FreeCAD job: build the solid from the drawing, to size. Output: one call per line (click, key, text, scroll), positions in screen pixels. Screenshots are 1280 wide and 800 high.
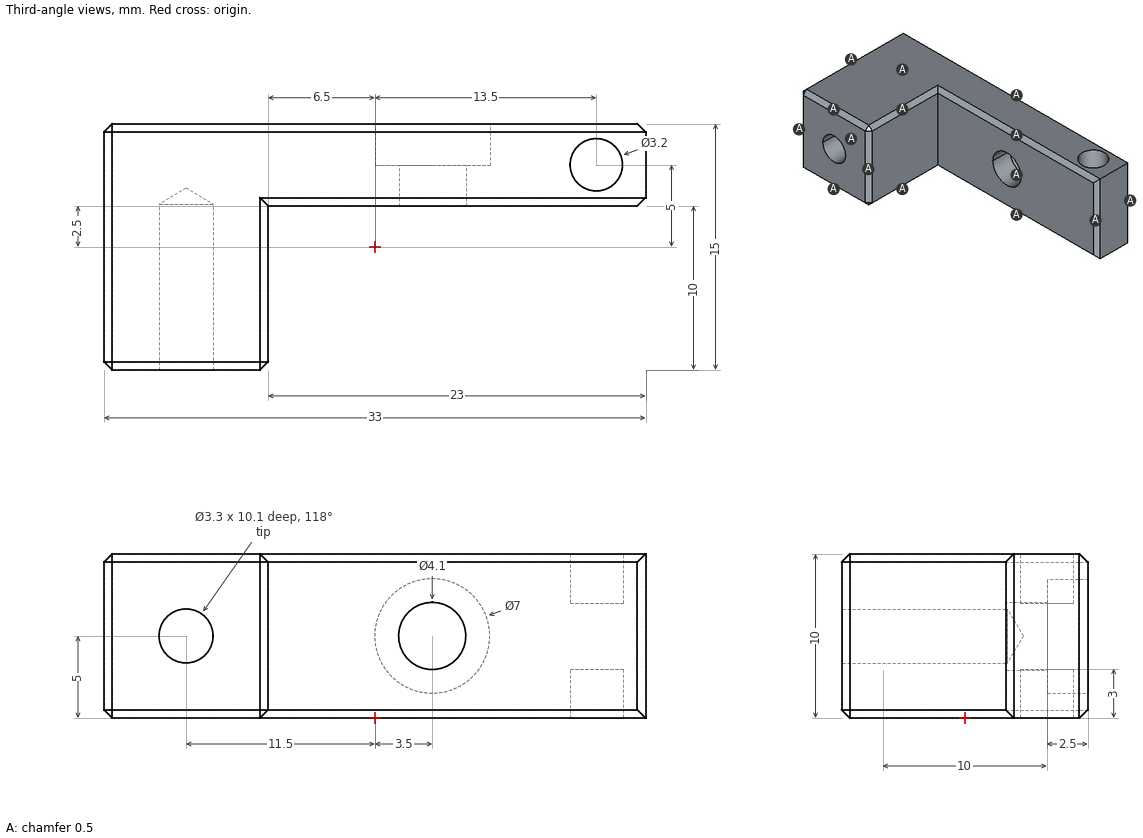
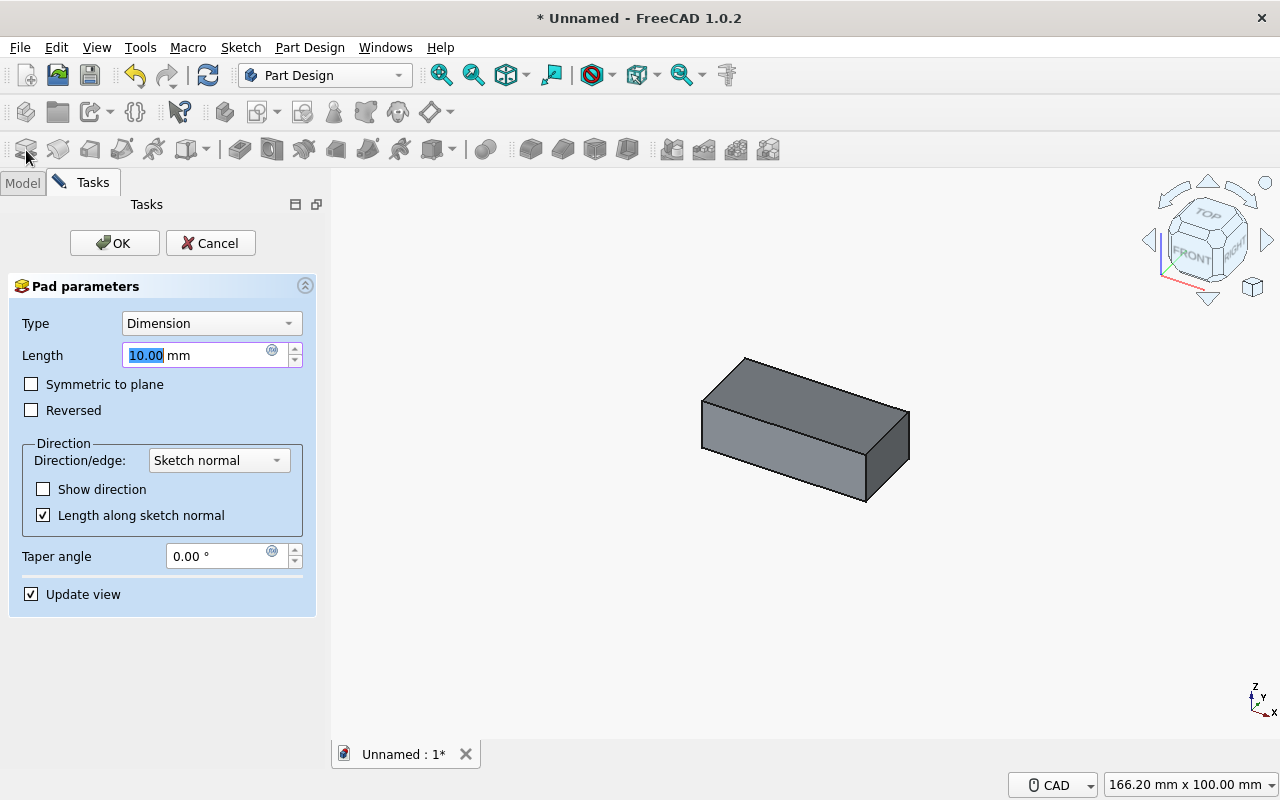
text(10)
key(Tab)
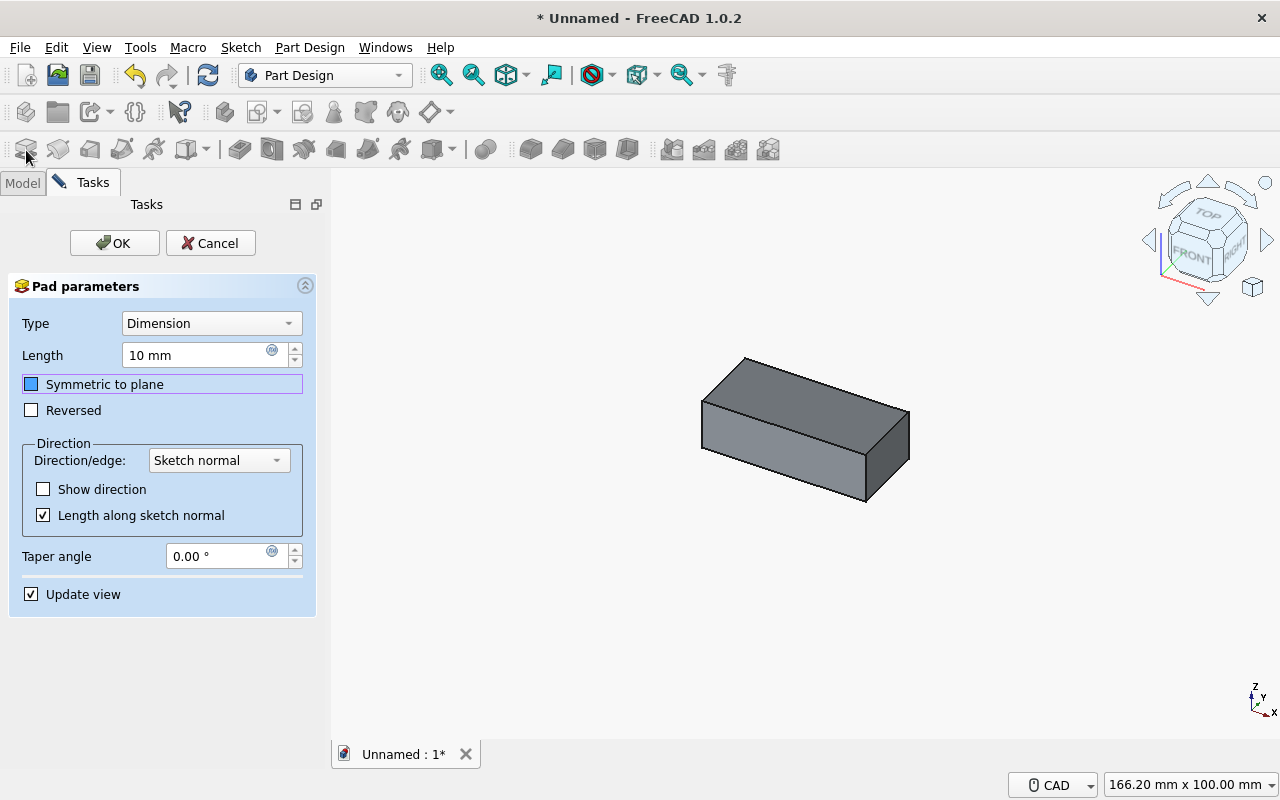
click(115, 243)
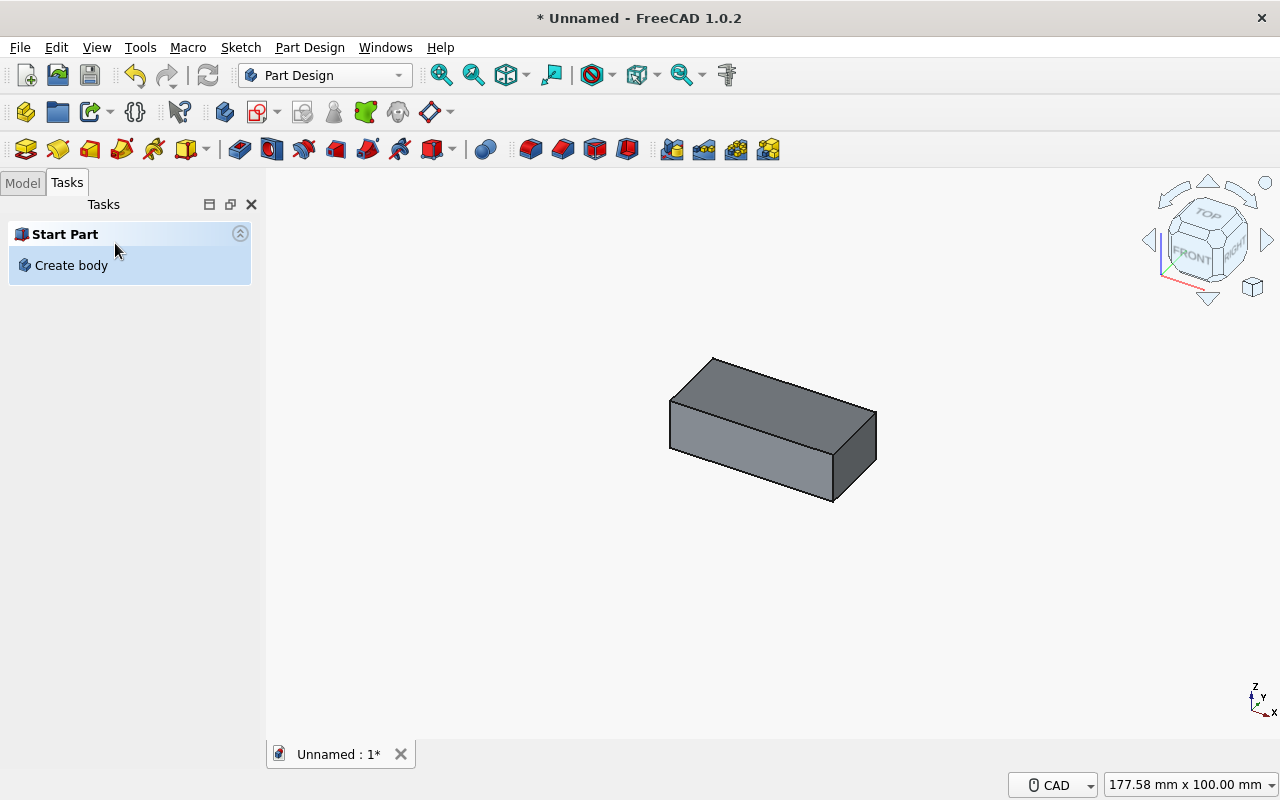
click(442, 76)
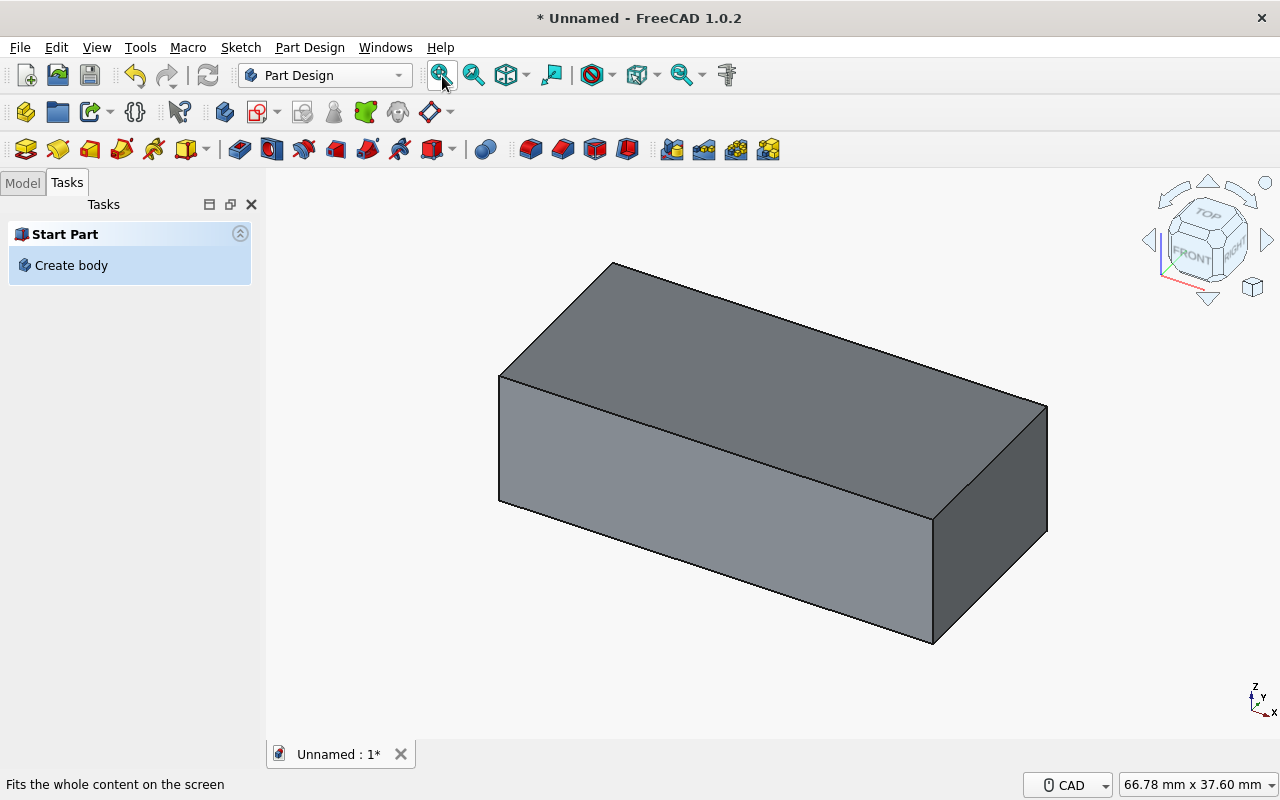
click(835, 411)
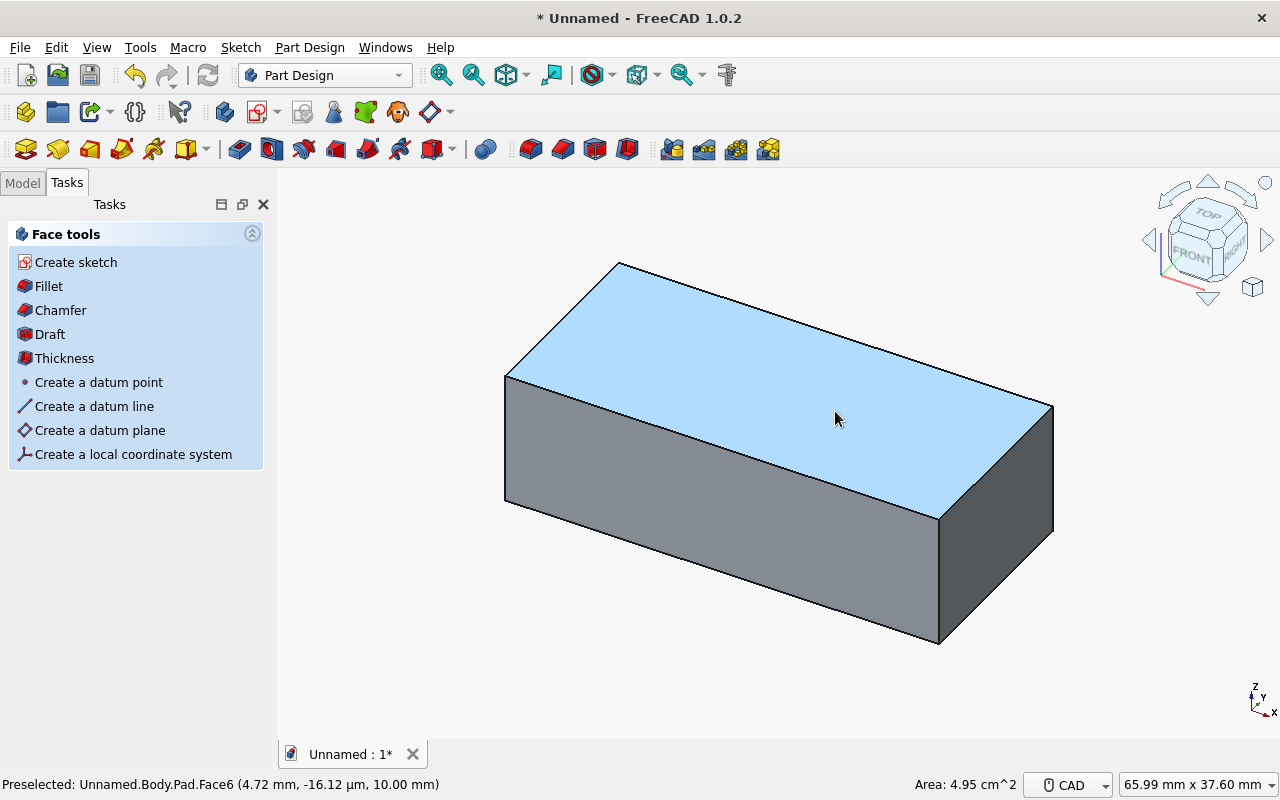
click(258, 112)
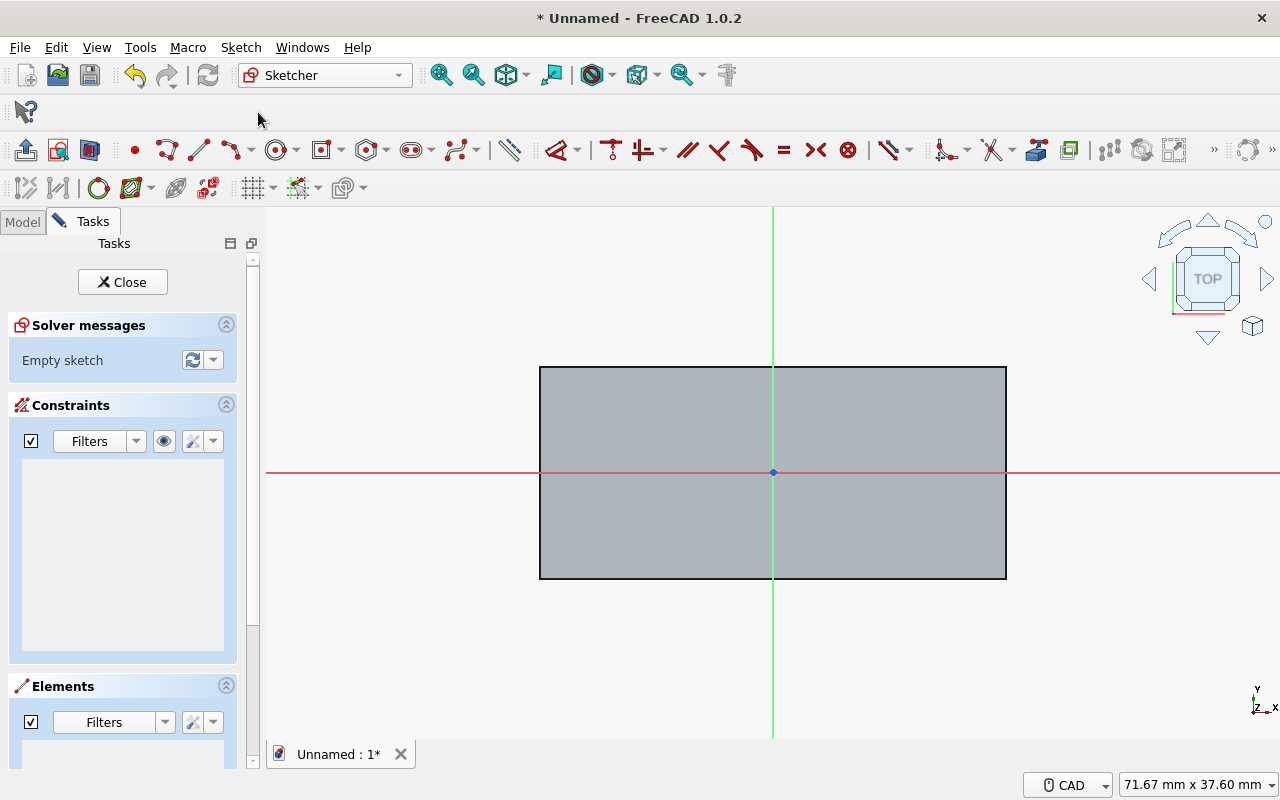
scroll(1013, 551, up, 3)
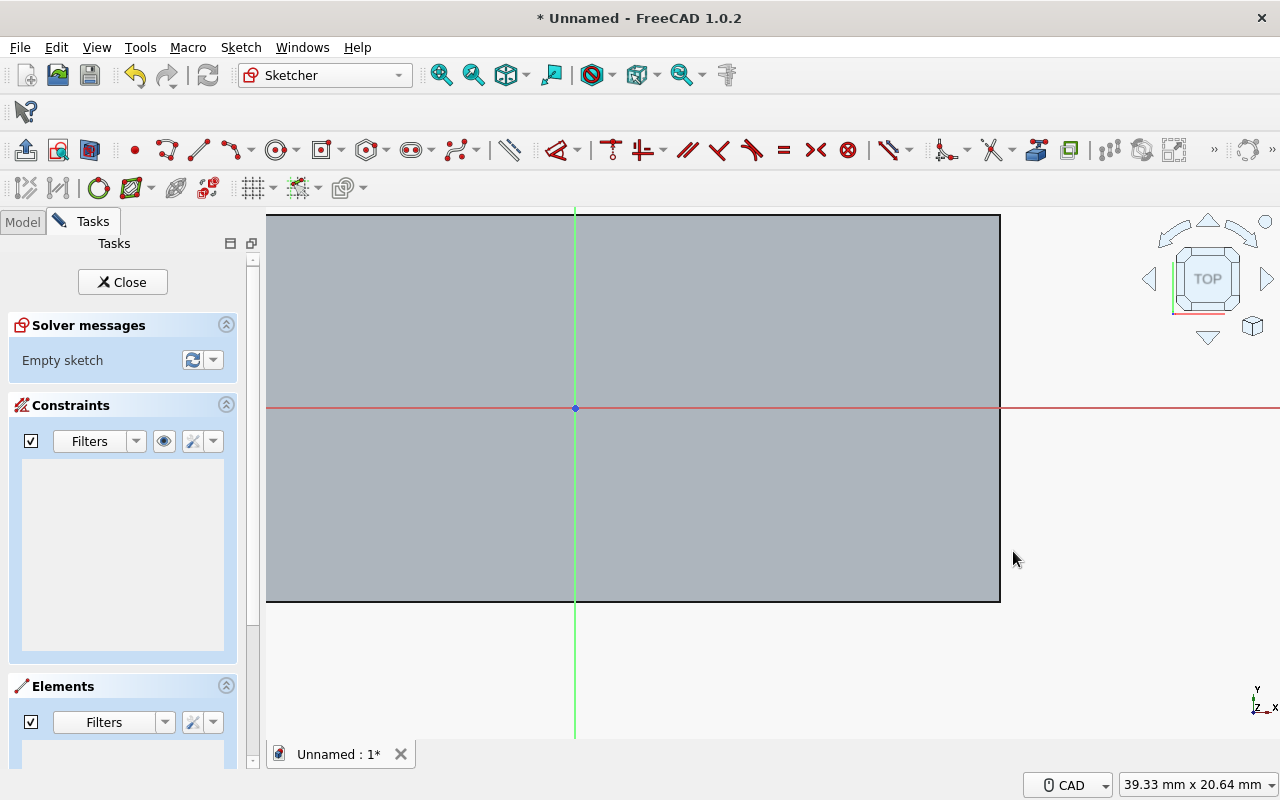
click(344, 150)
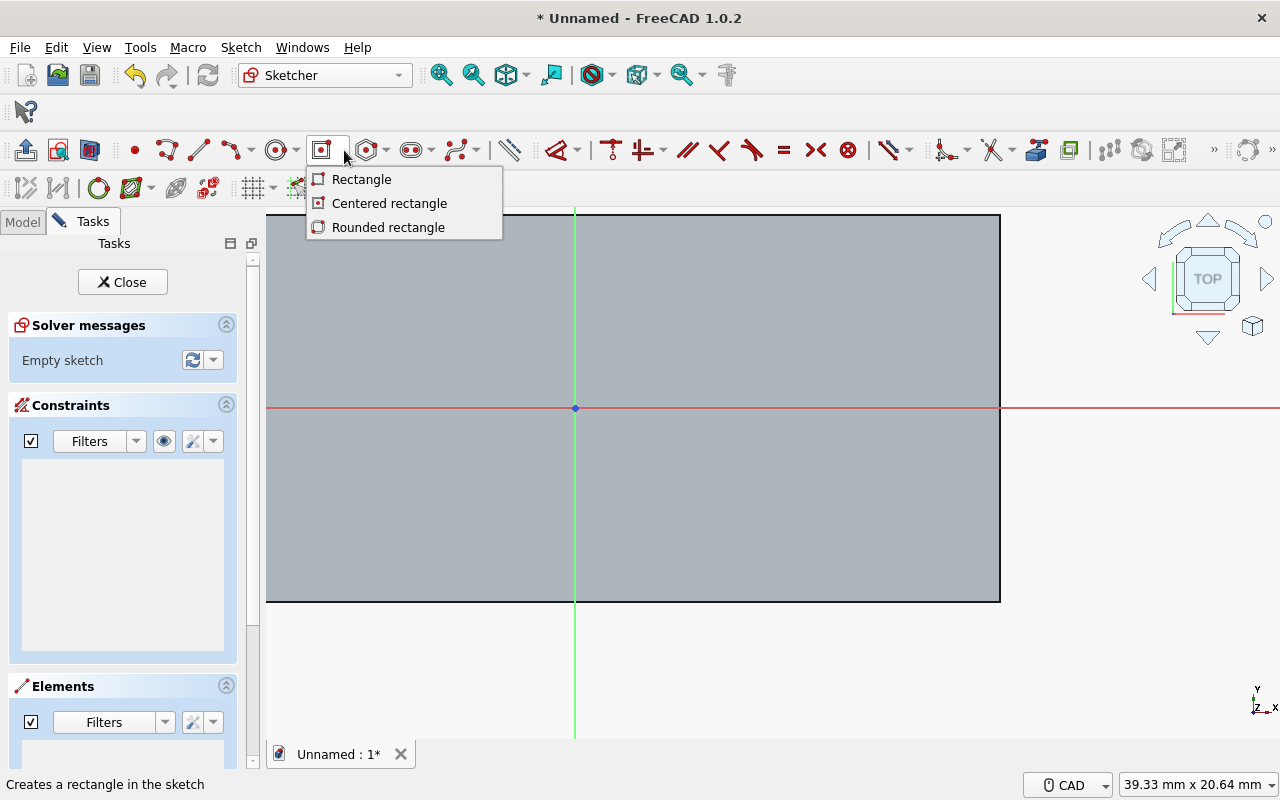
click(404, 179)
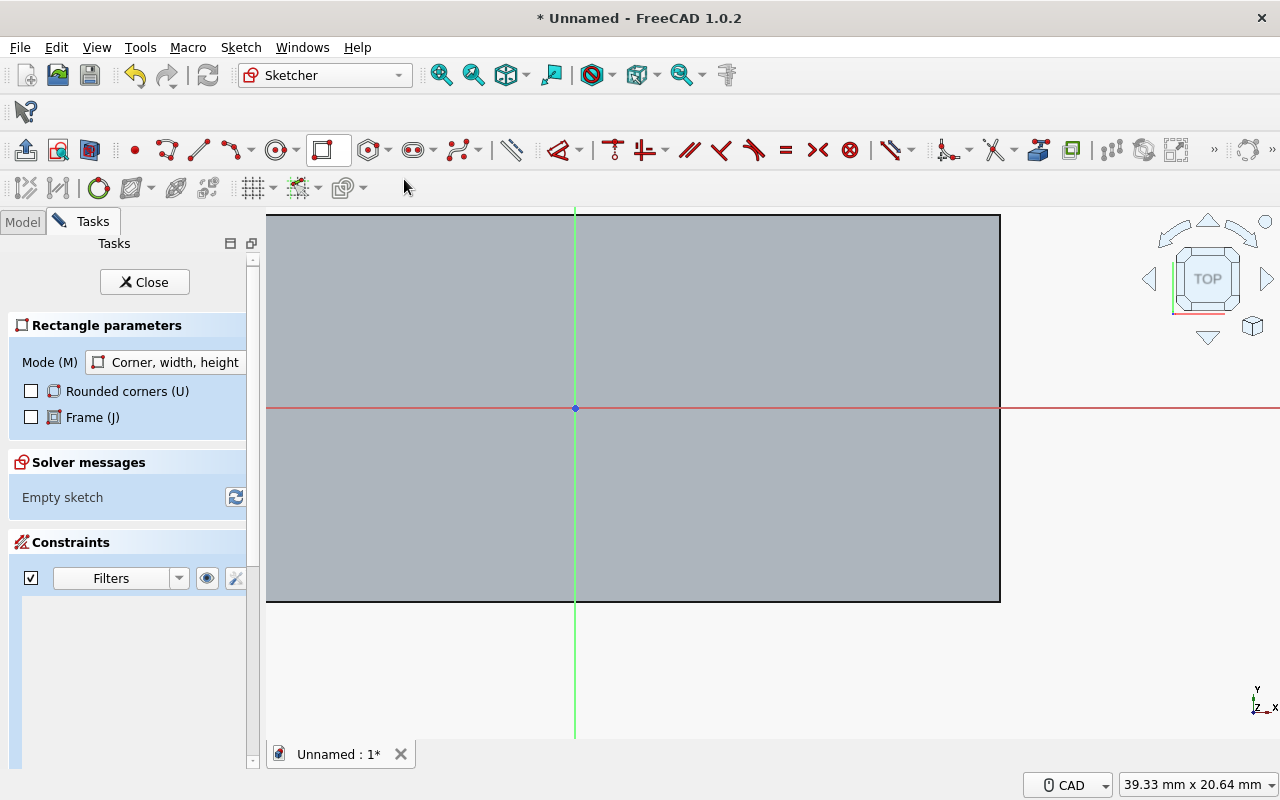
click(408, 344)
move(1000, 602)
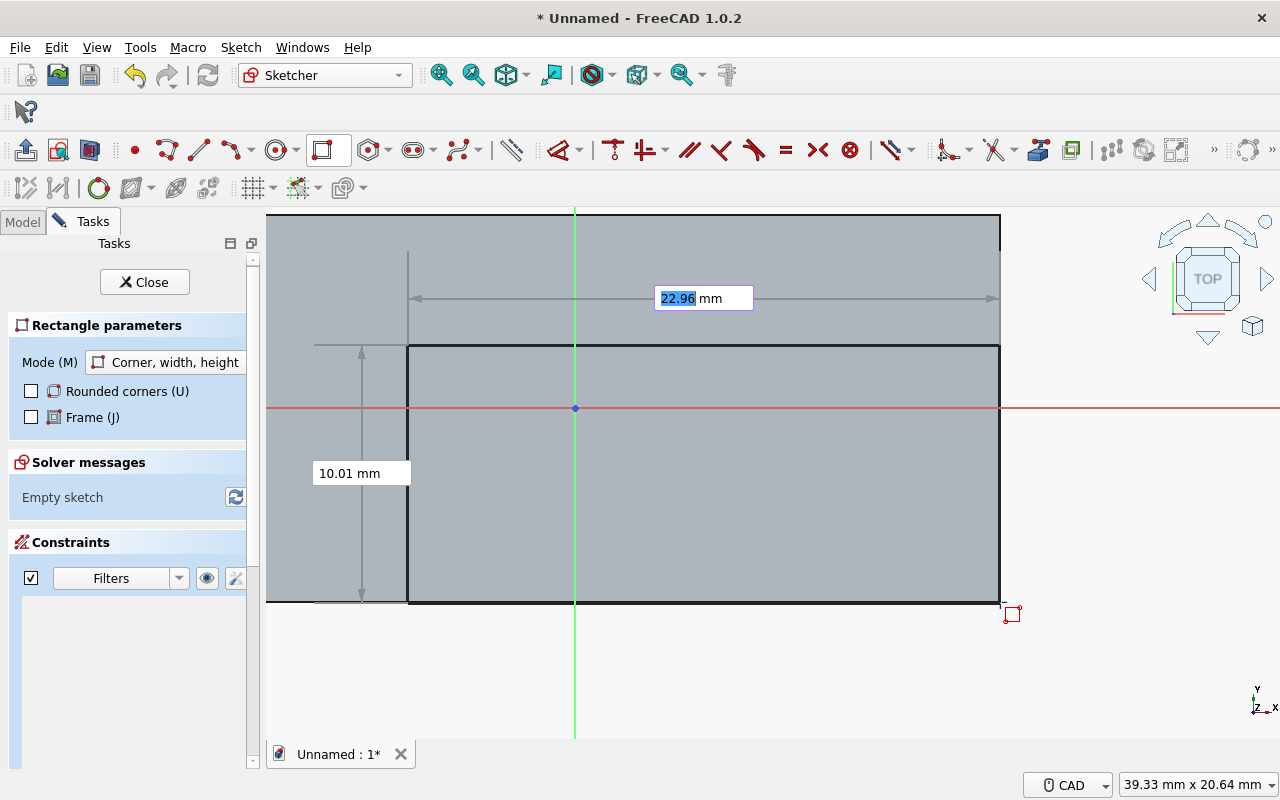
text(23)
key(Tab)
text(10)
key(Return)
key(Escape)